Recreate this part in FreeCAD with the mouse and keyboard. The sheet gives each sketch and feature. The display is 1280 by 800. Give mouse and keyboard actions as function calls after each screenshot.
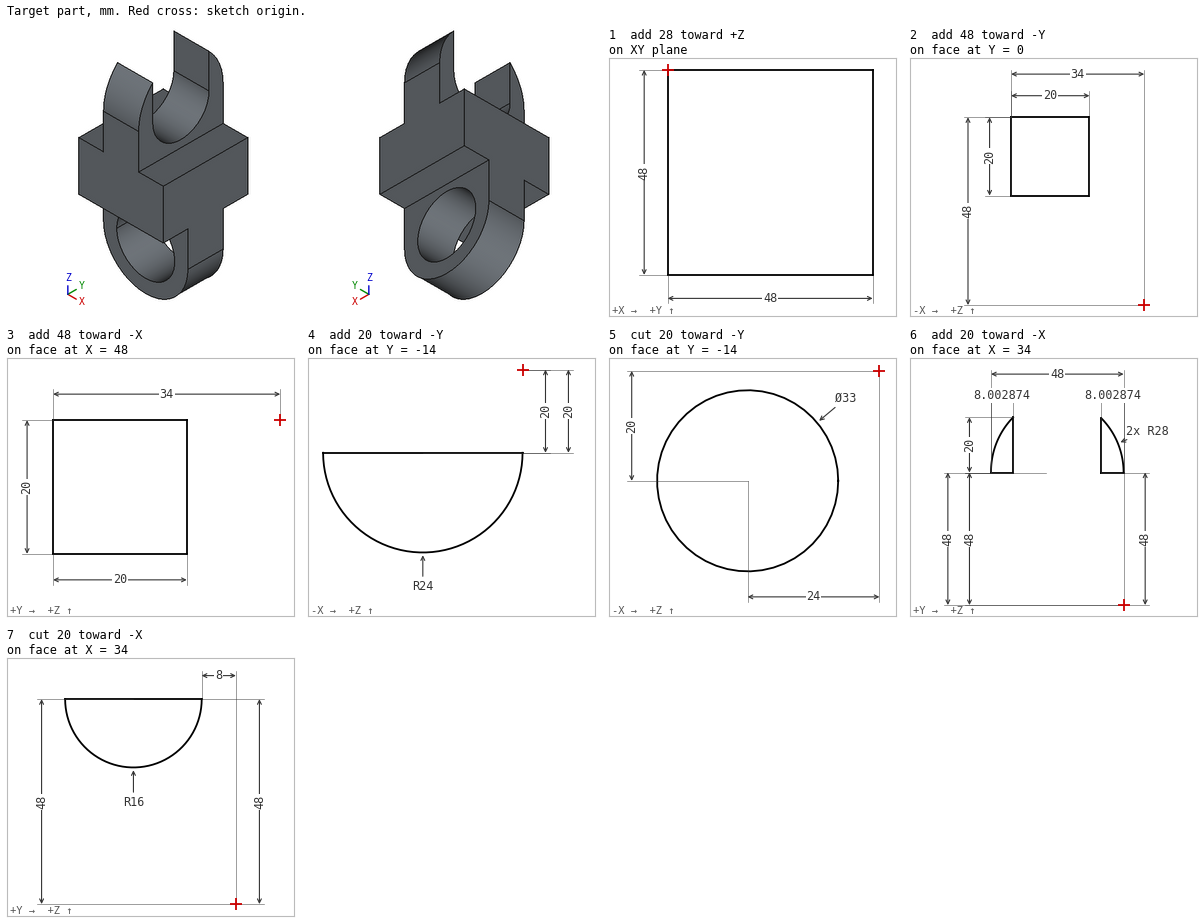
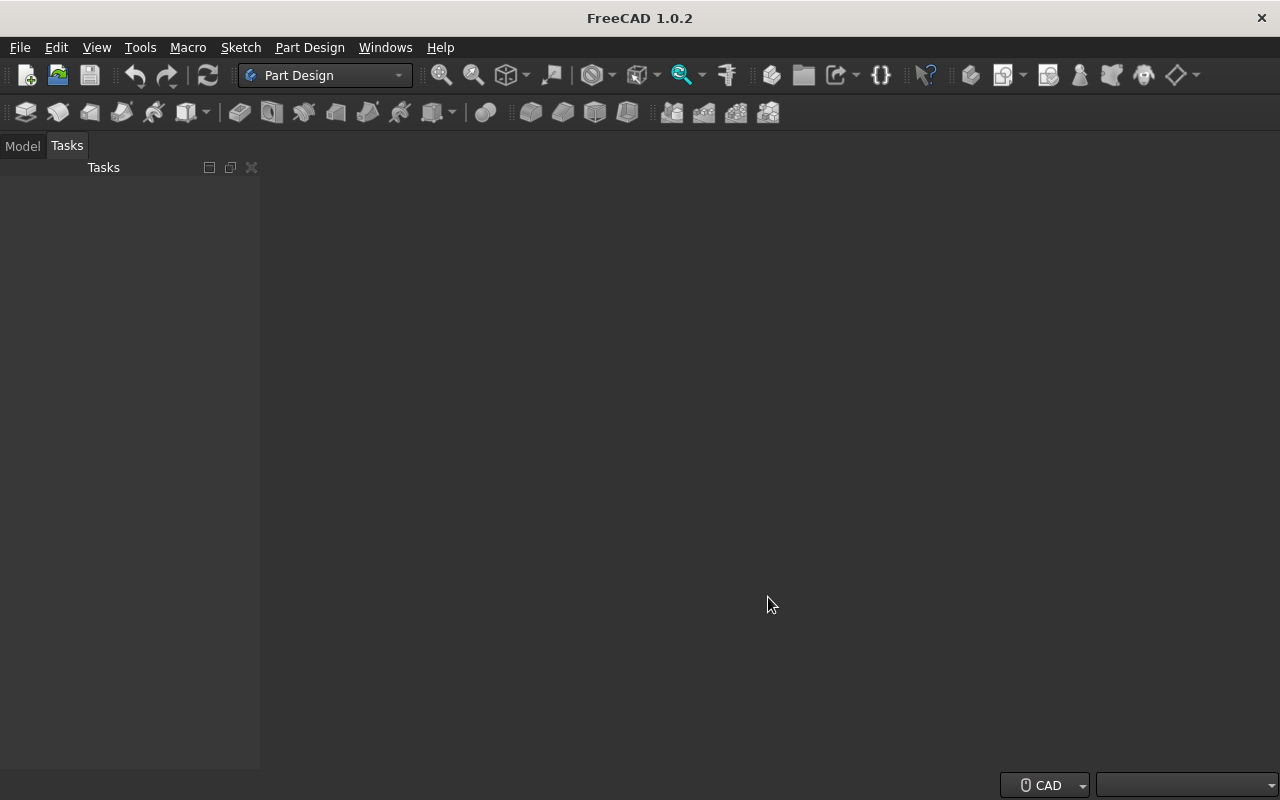
key(ctrl+n)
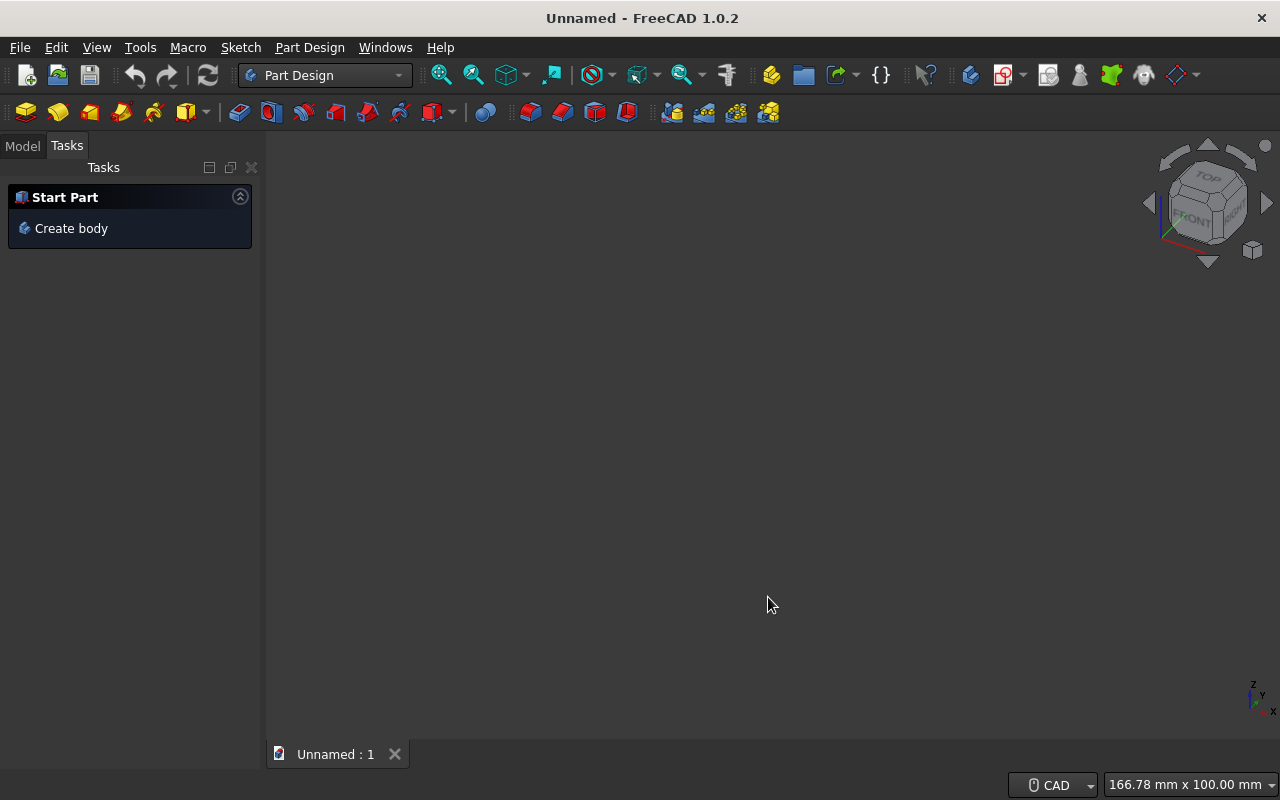
click(1004, 76)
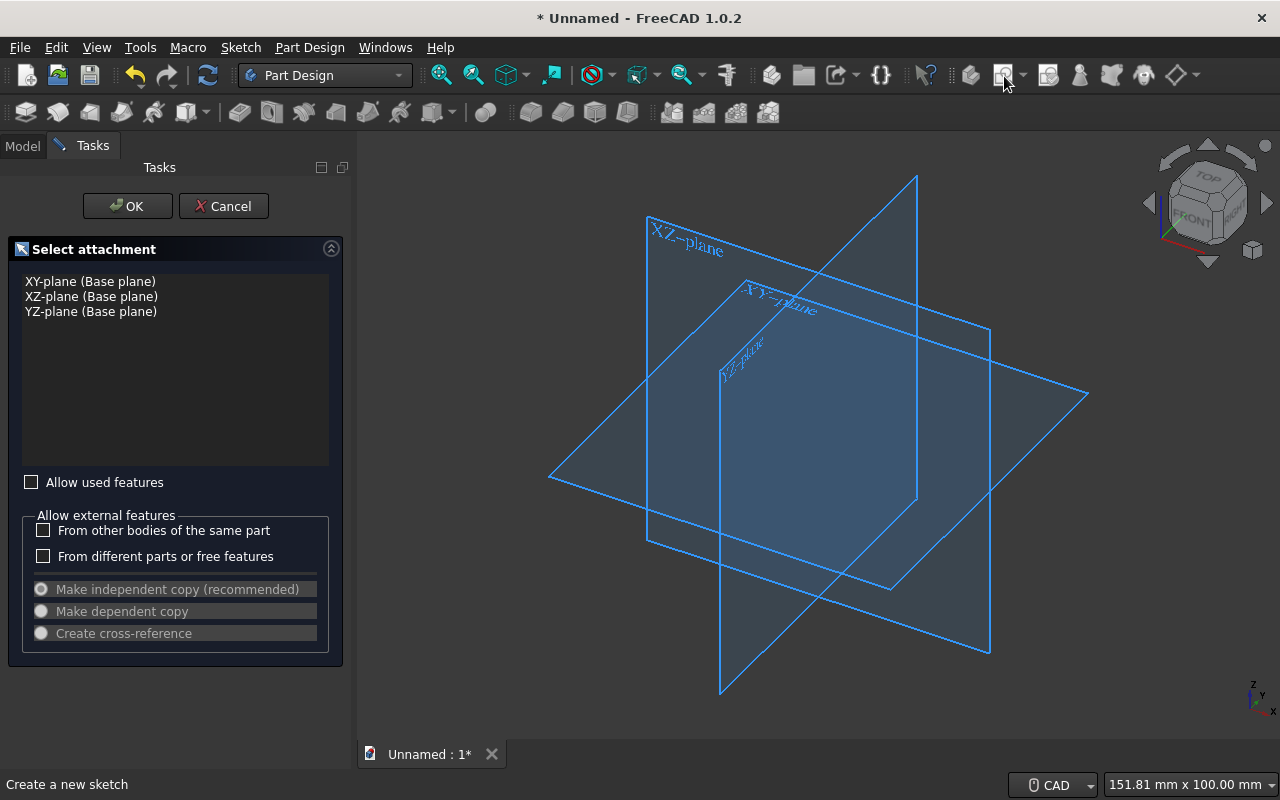
click(82, 282)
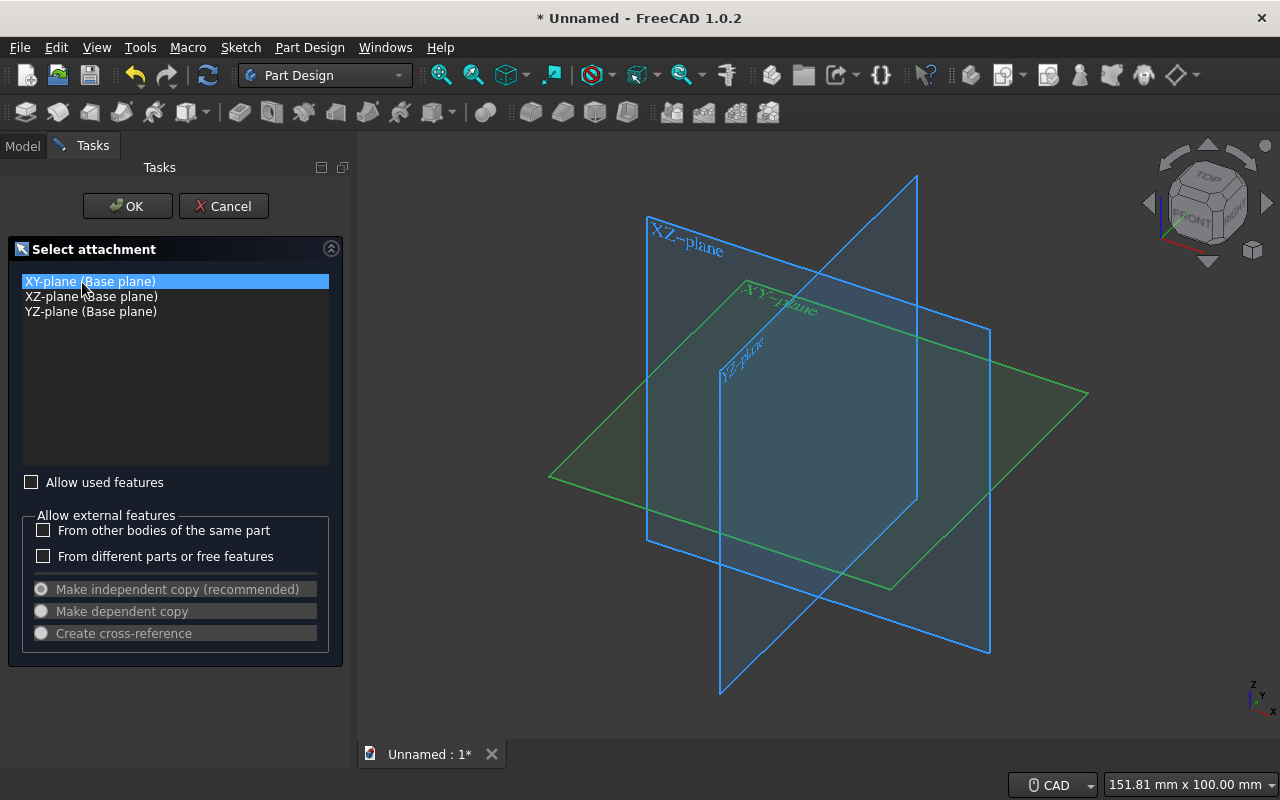
click(128, 206)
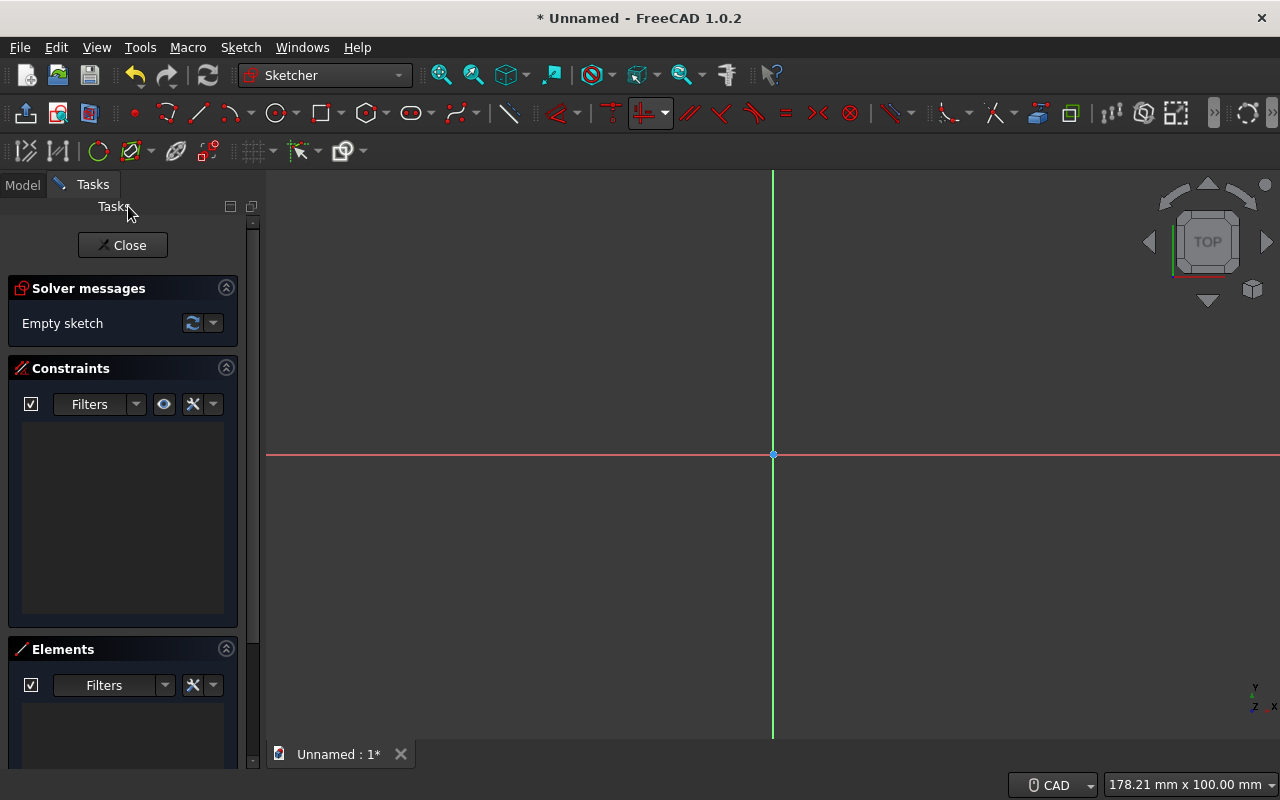
scroll(294, 198, down, 1)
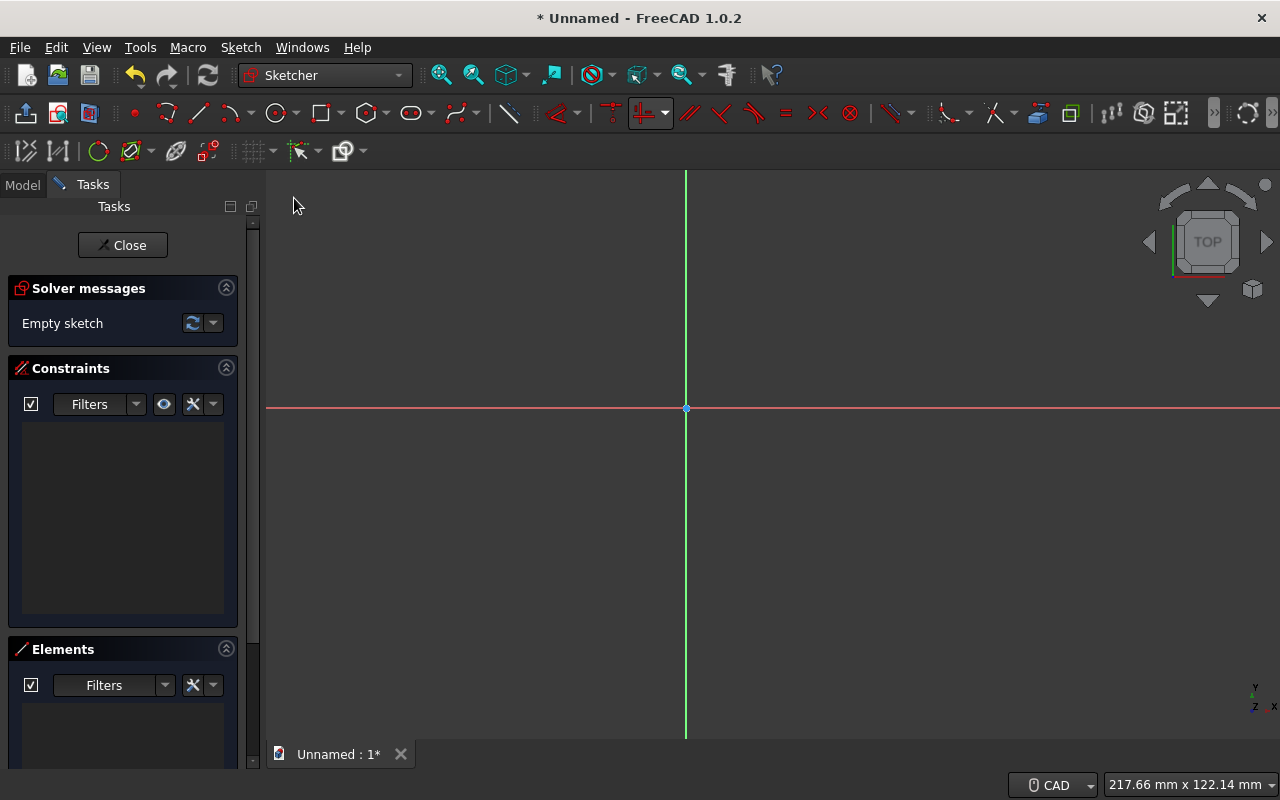
scroll(988, 653, up, 2)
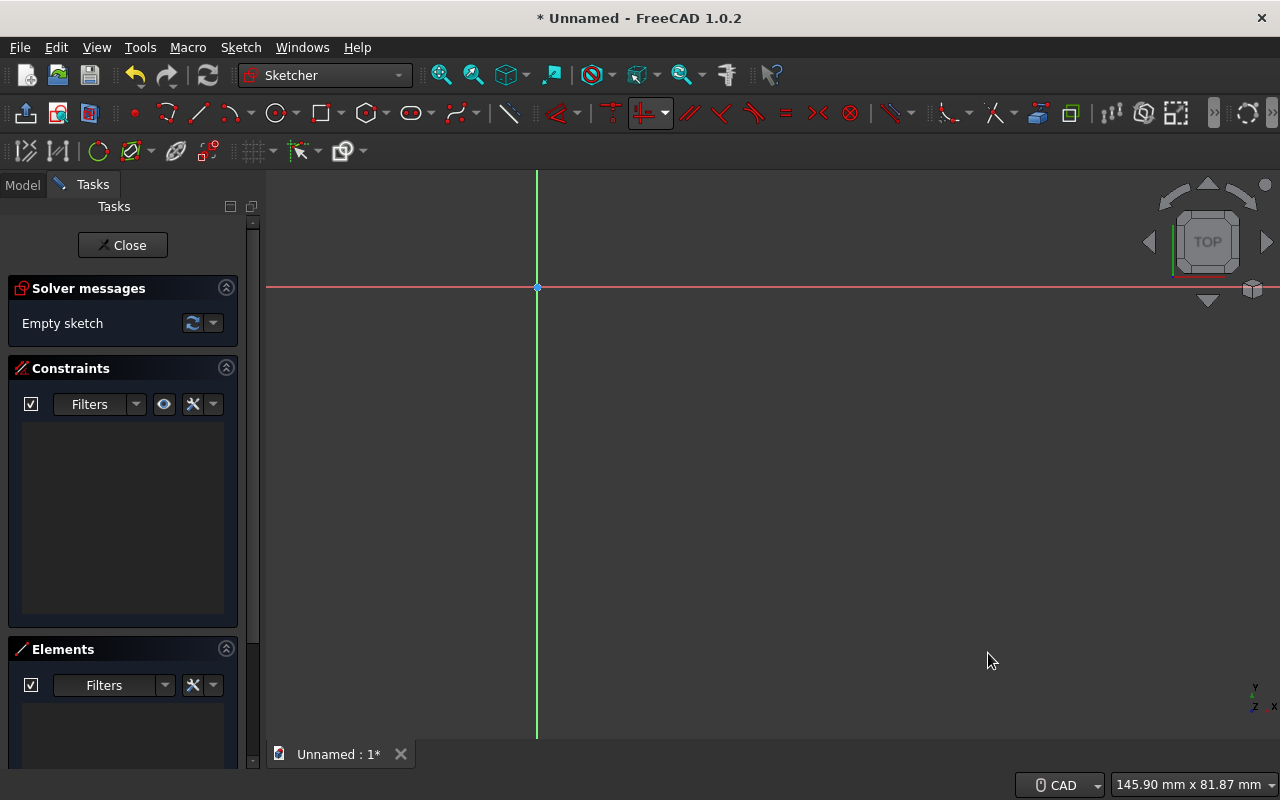
key(g)
key(r)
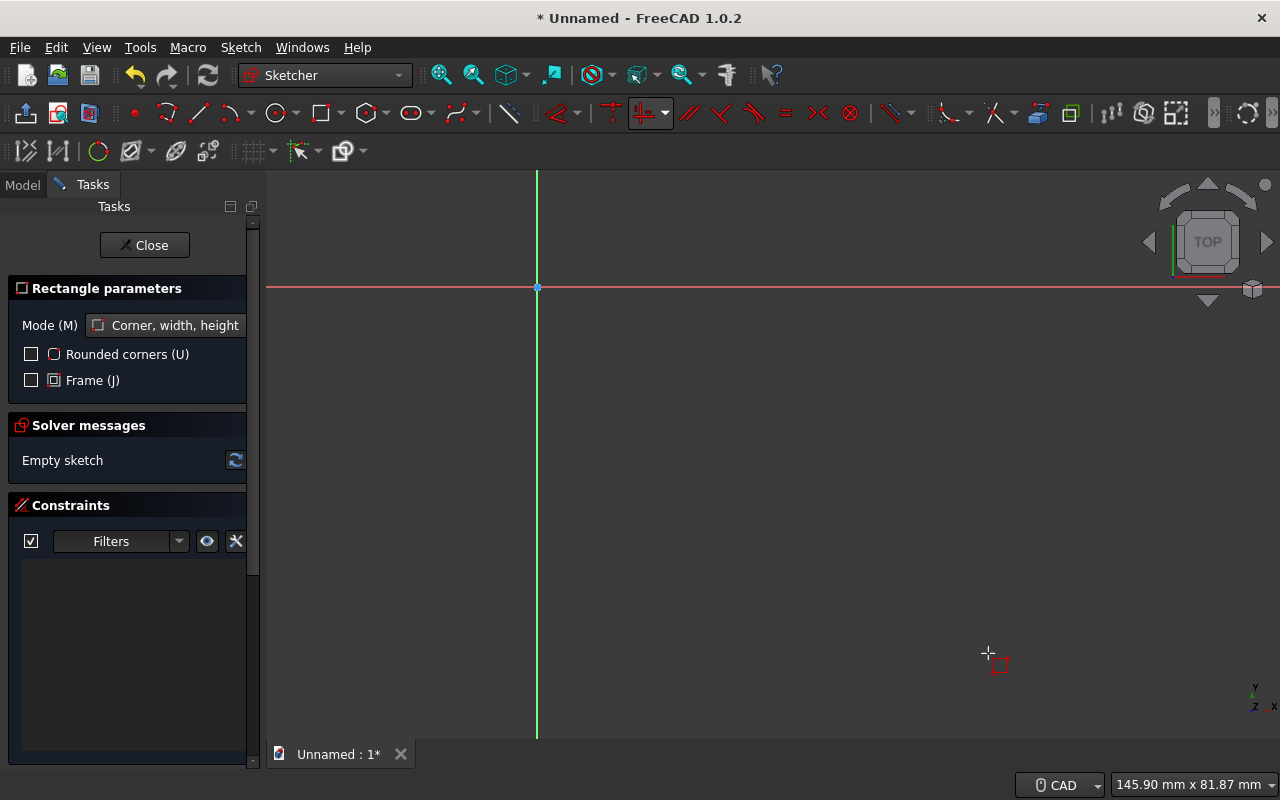
click(537, 287)
click(871, 621)
key(Escape)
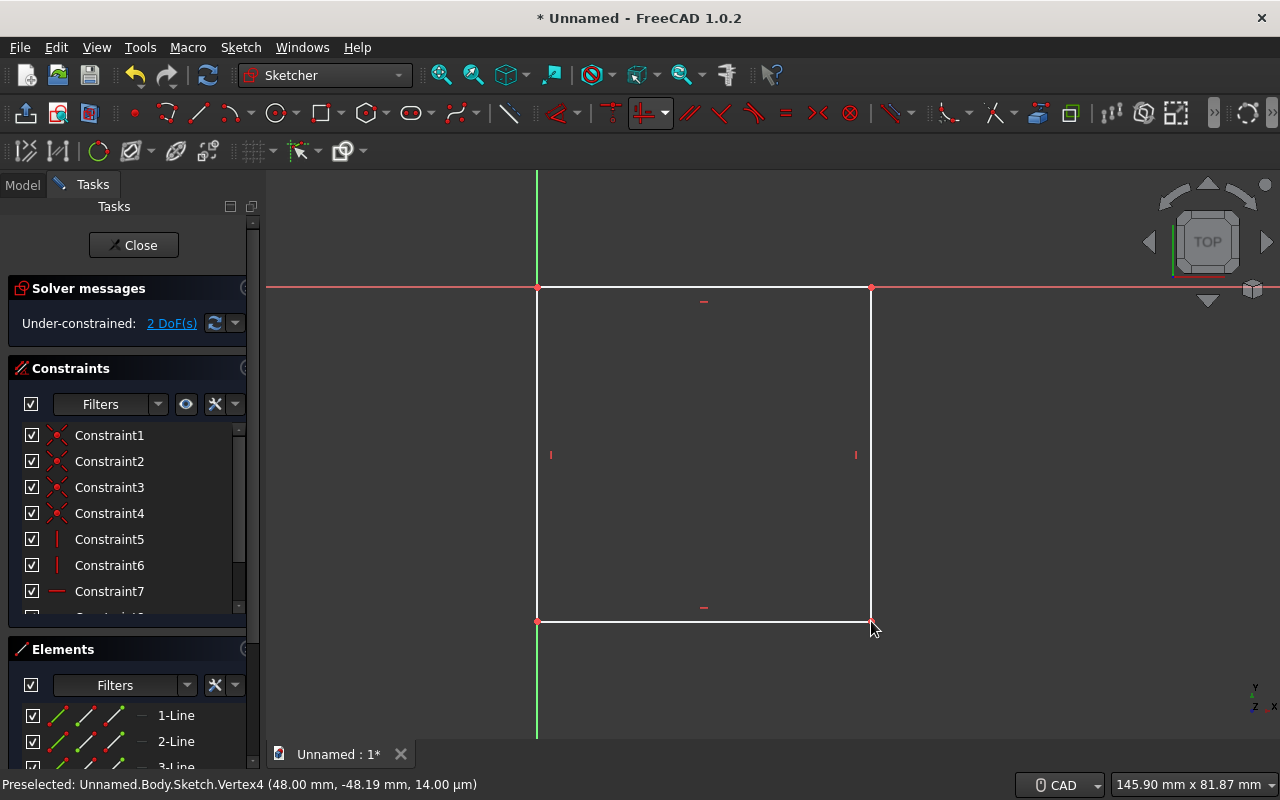
key(d)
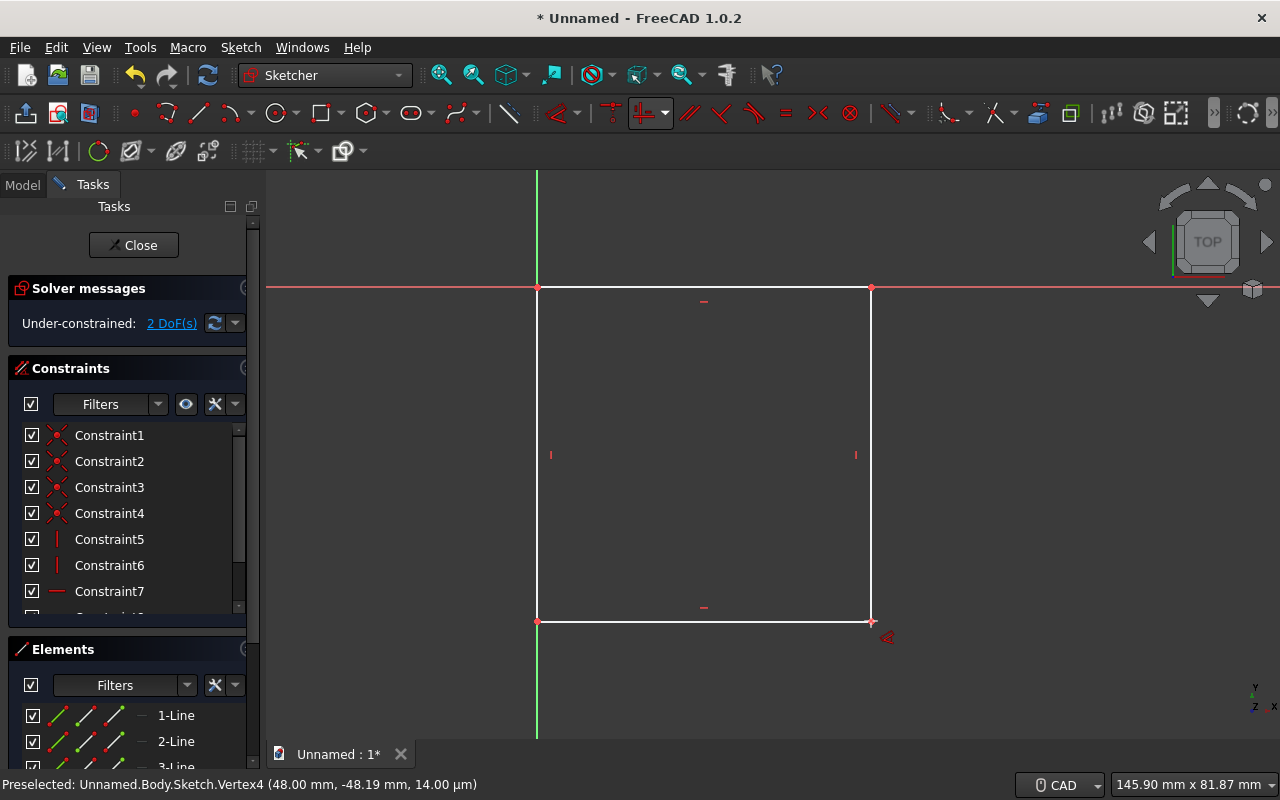
click(537, 388)
click(503, 455)